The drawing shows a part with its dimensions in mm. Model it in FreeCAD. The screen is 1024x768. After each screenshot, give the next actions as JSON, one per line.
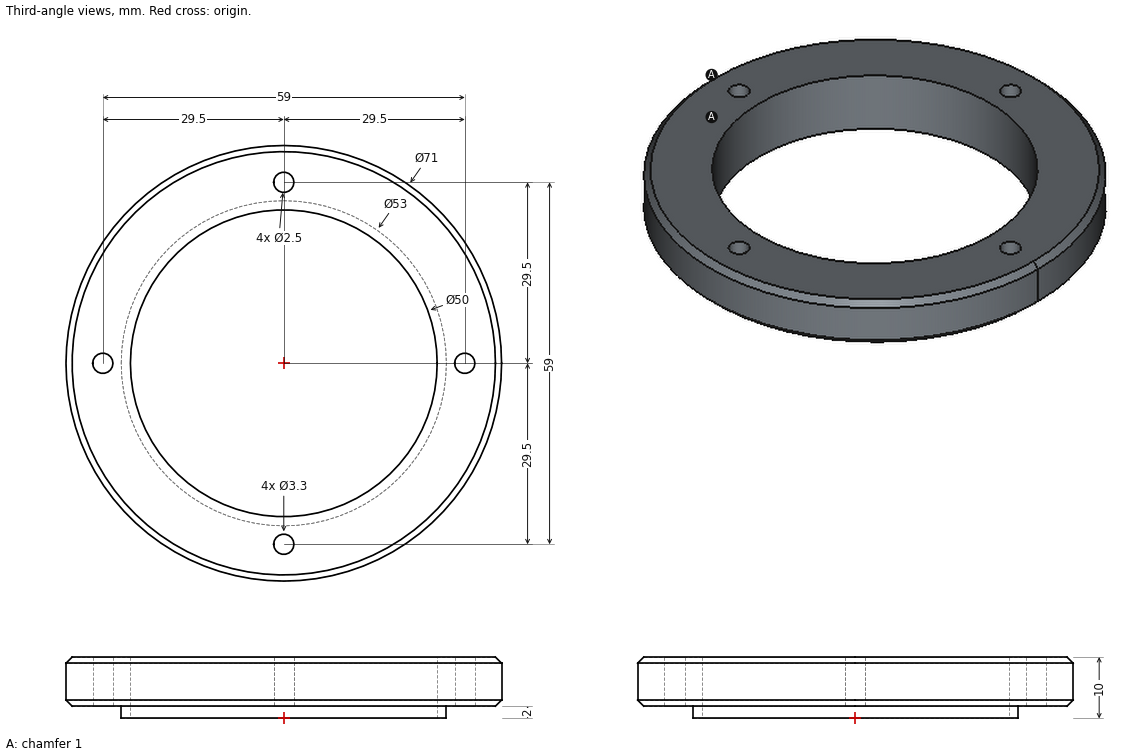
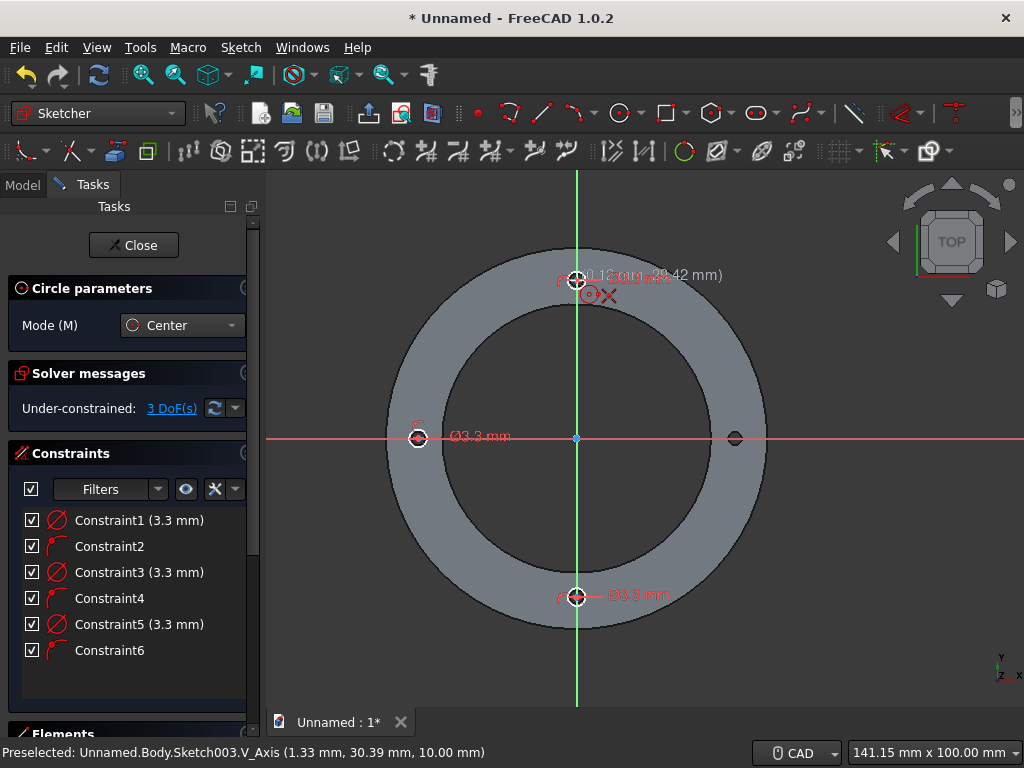
{"action": "scroll", "coordinate": [735, 438], "scroll_direction": "up", "scroll_amount": 5}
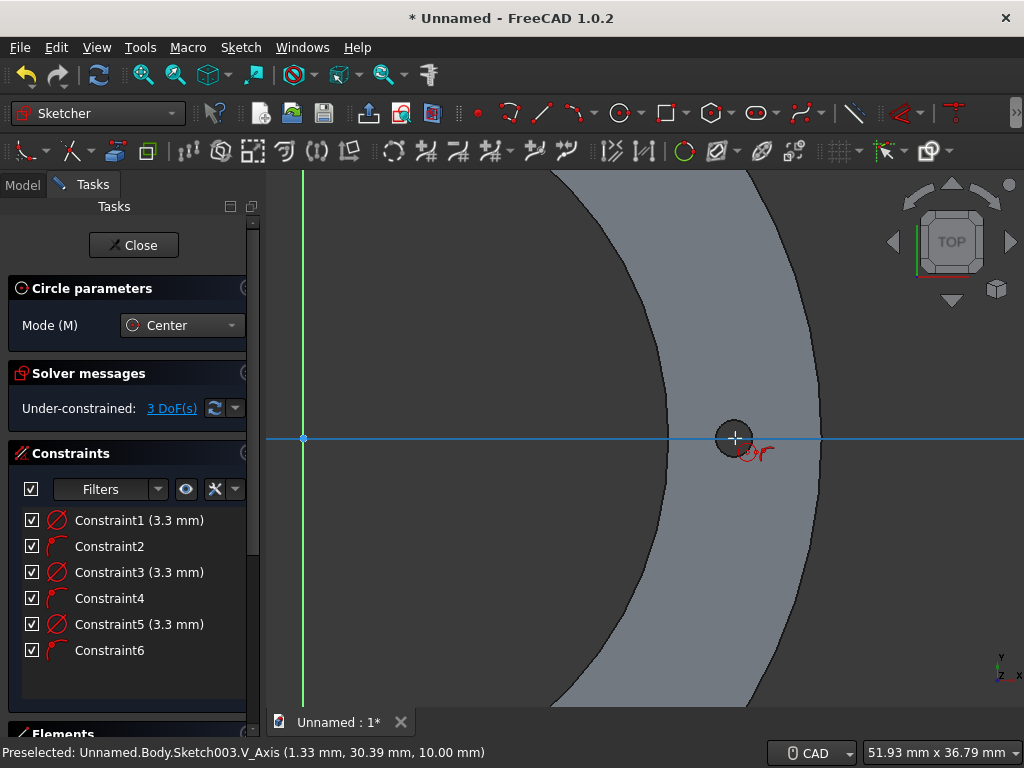
{"action": "left_click", "coordinate": [734, 438]}
{"action": "mouse_move", "coordinate": [751, 421]}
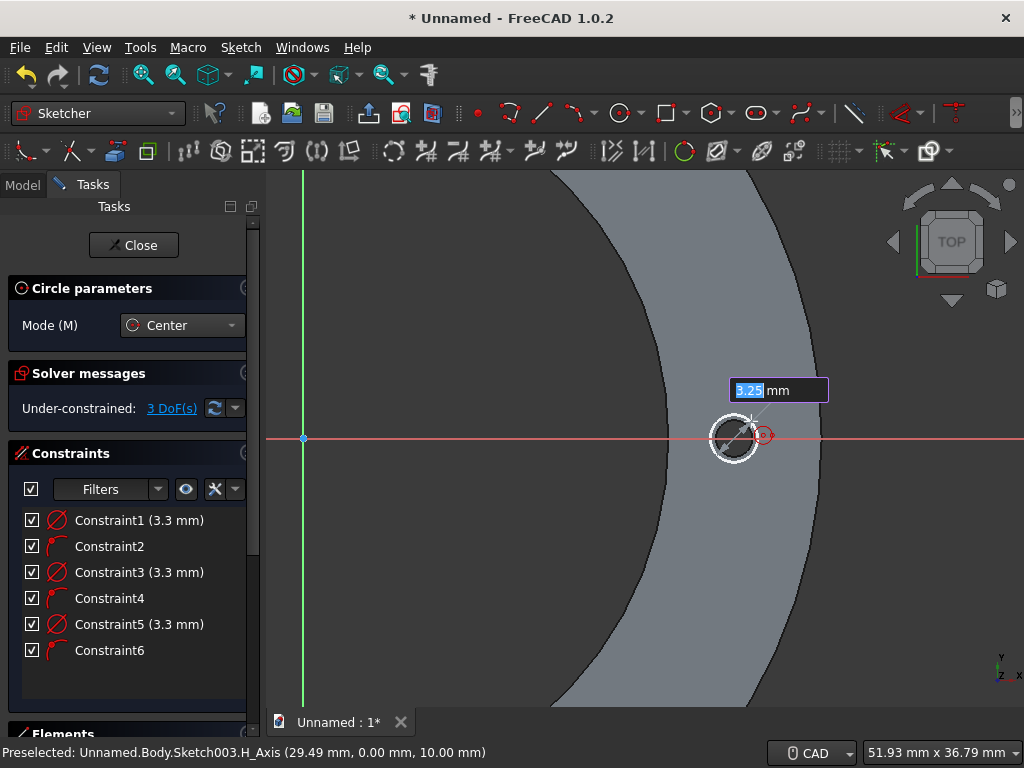
{"action": "type", "text": "3.3"}
{"action": "key", "text": "Return"}
{"action": "key", "text": "Escape"}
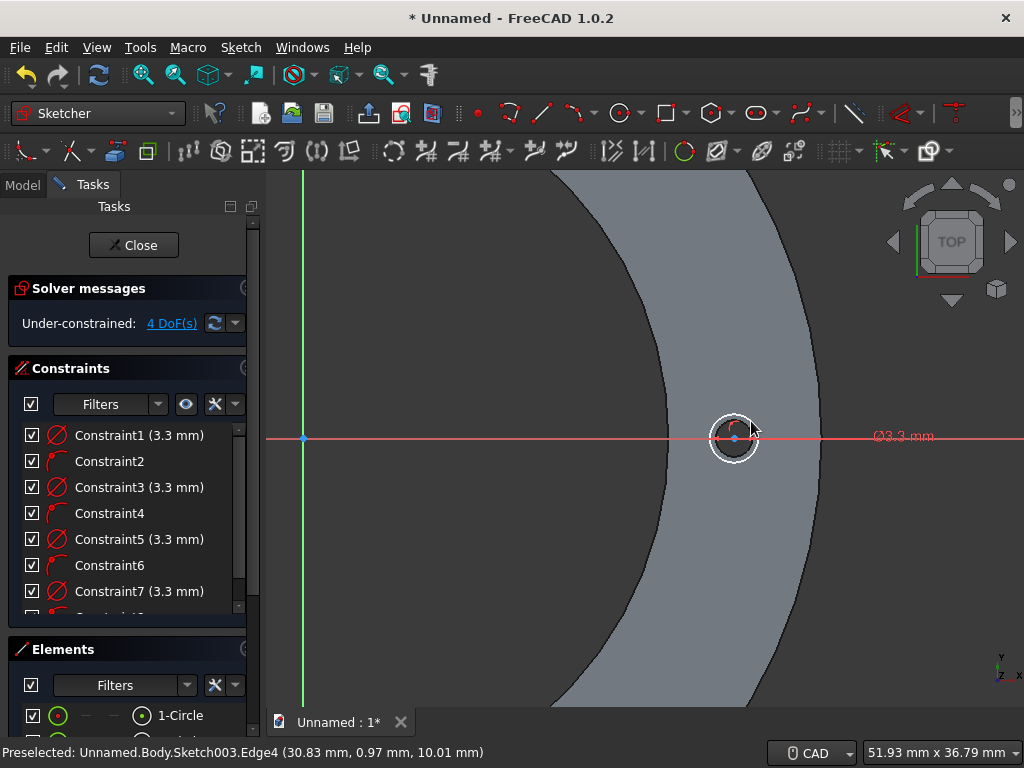
{"action": "scroll", "coordinate": [735, 439], "scroll_direction": "down", "scroll_amount": 5}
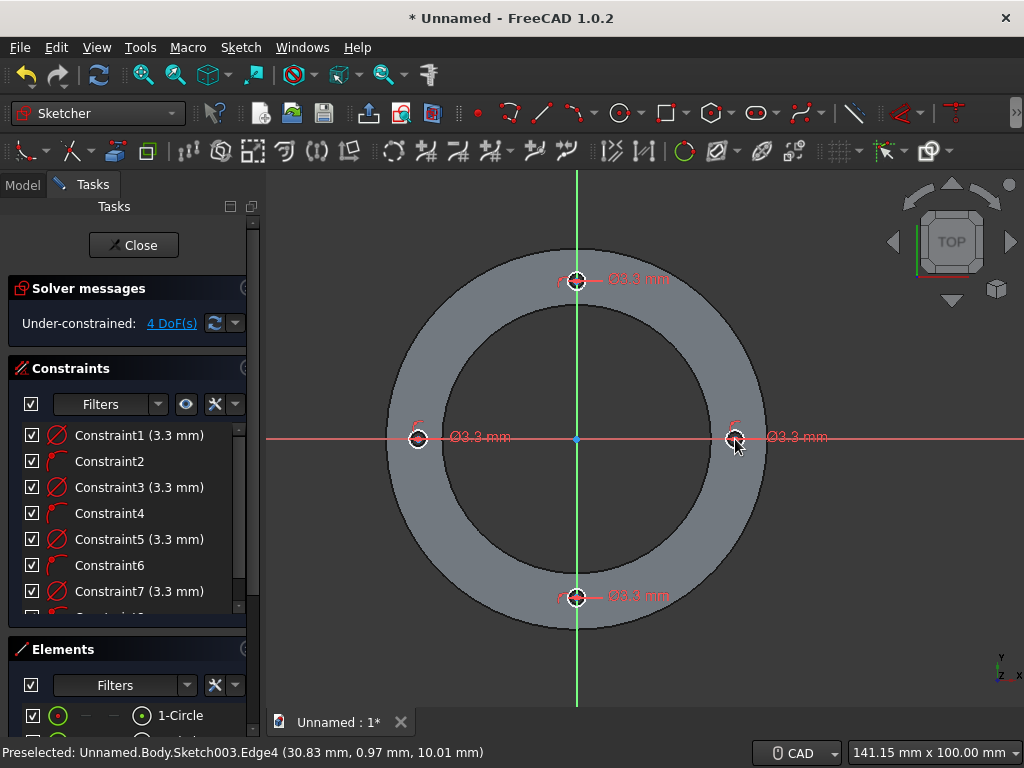
{"action": "left_click", "coordinate": [577, 598]}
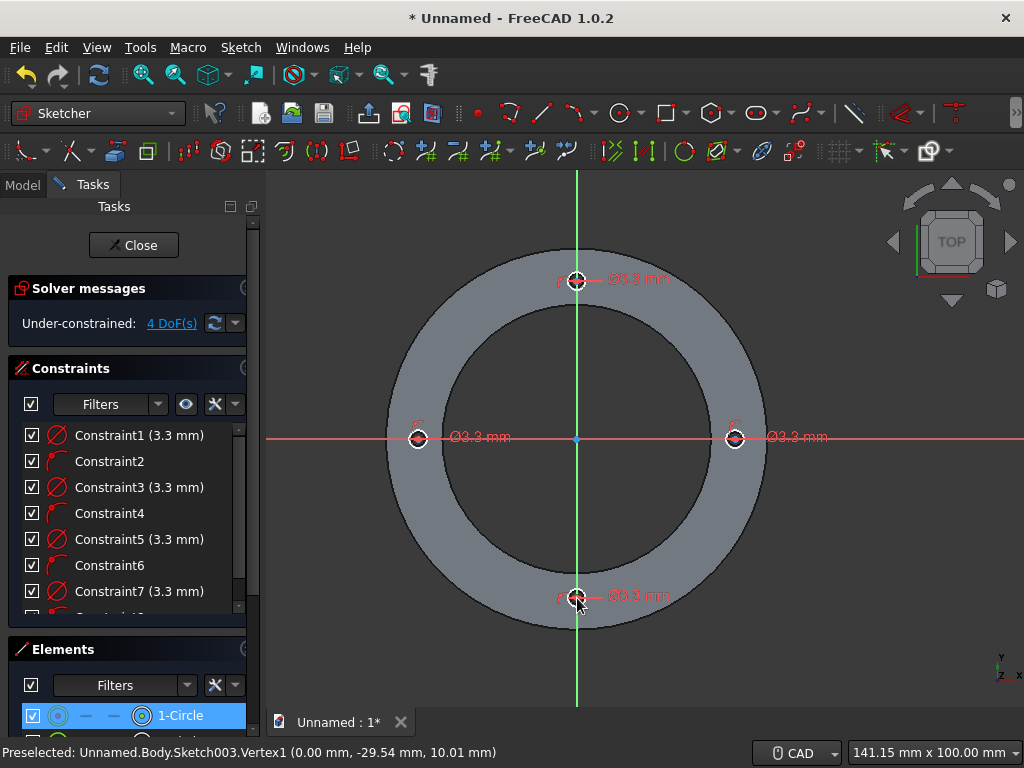
{"action": "left_click", "coordinate": [577, 281]}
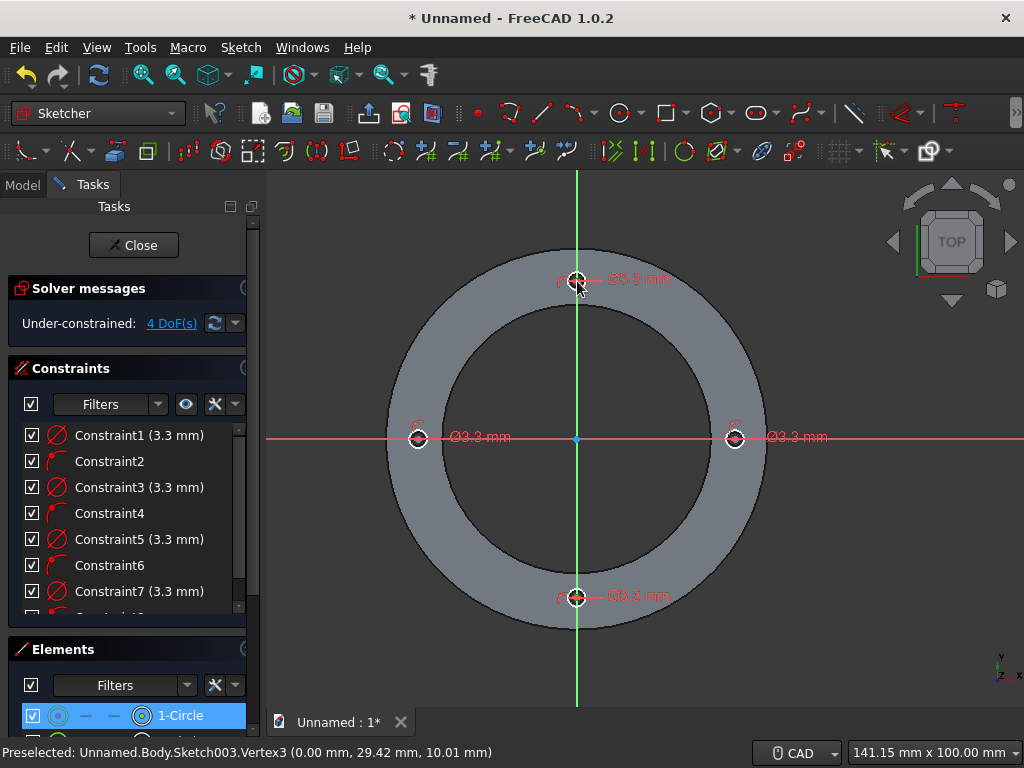
{"action": "key", "text": "i"}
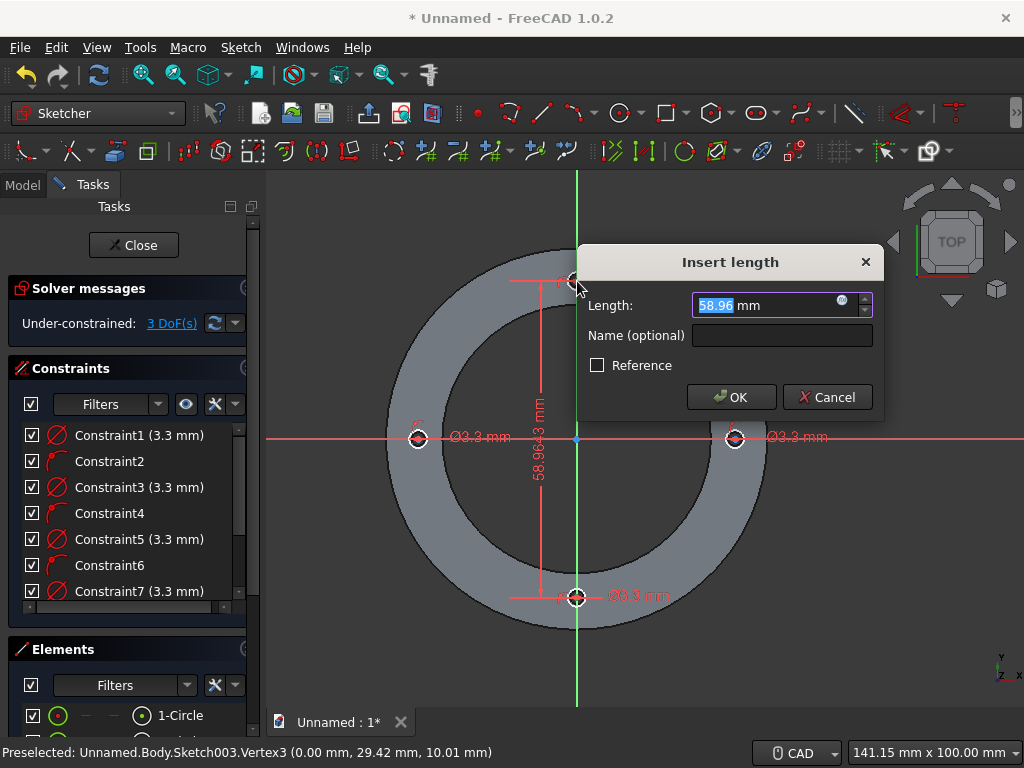
{"action": "type", "text": "59"}
{"action": "key", "text": "Return"}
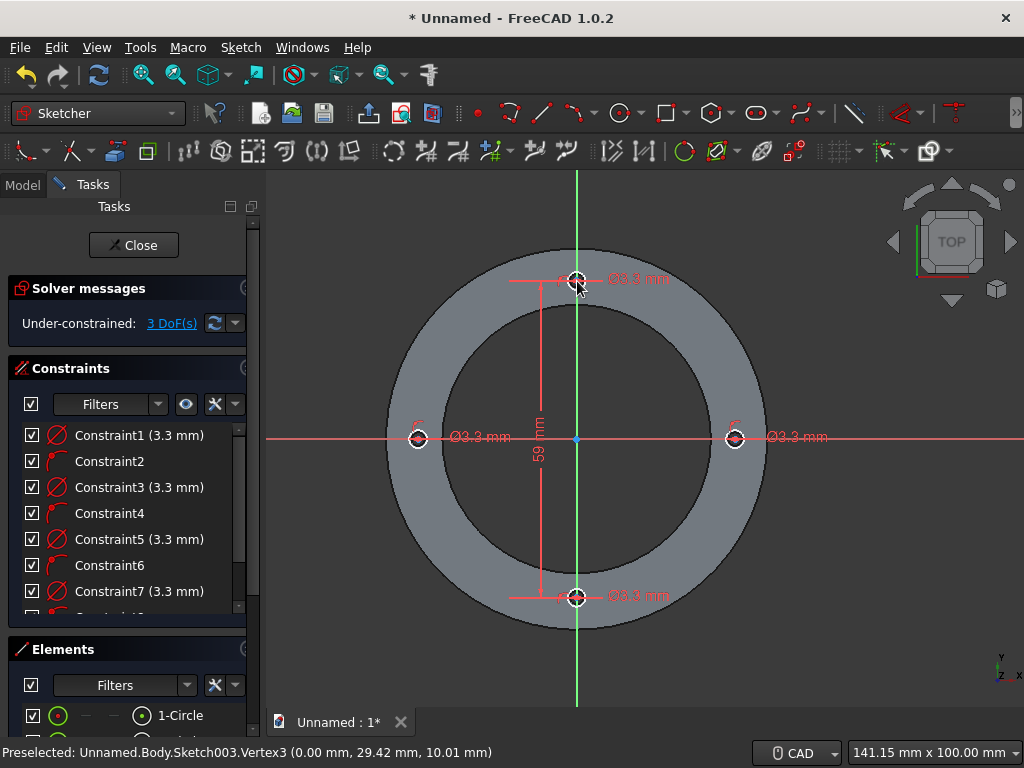
{"action": "left_click", "coordinate": [418, 439]}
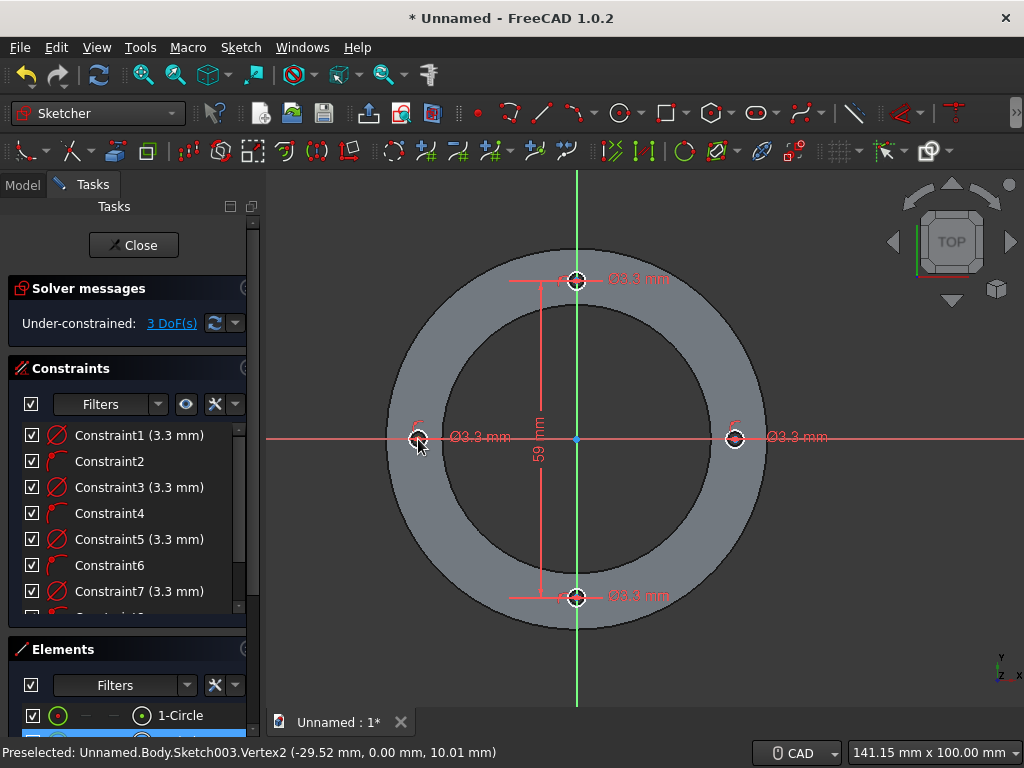
{"action": "left_click", "coordinate": [735, 439]}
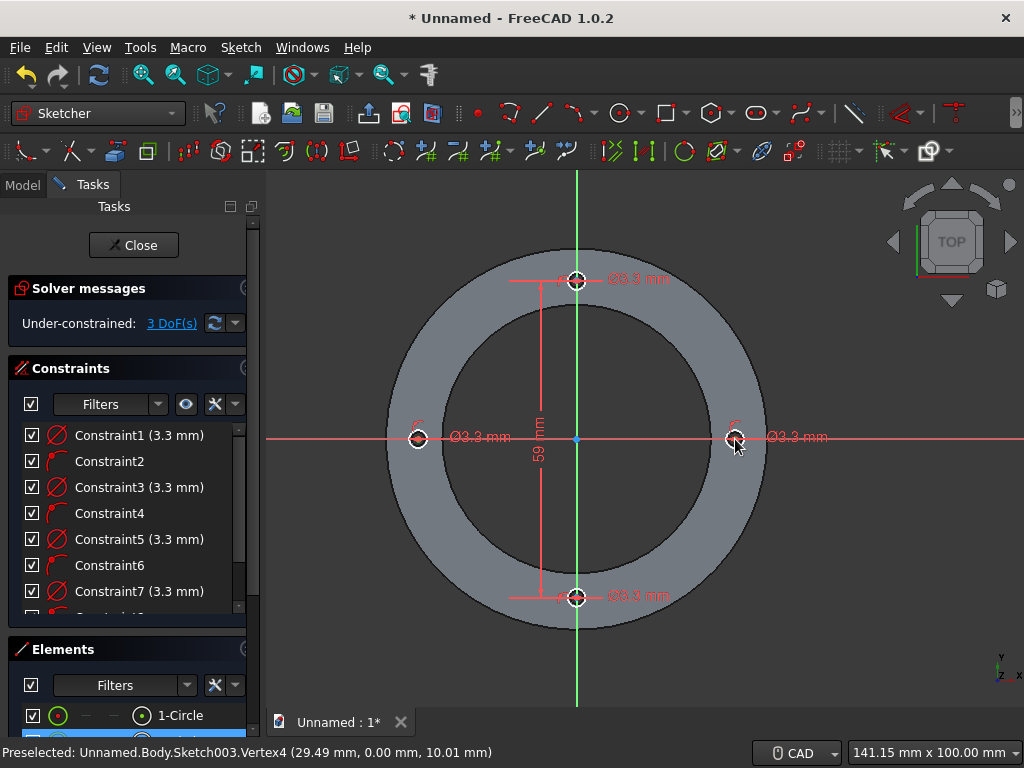
{"action": "key", "text": "l"}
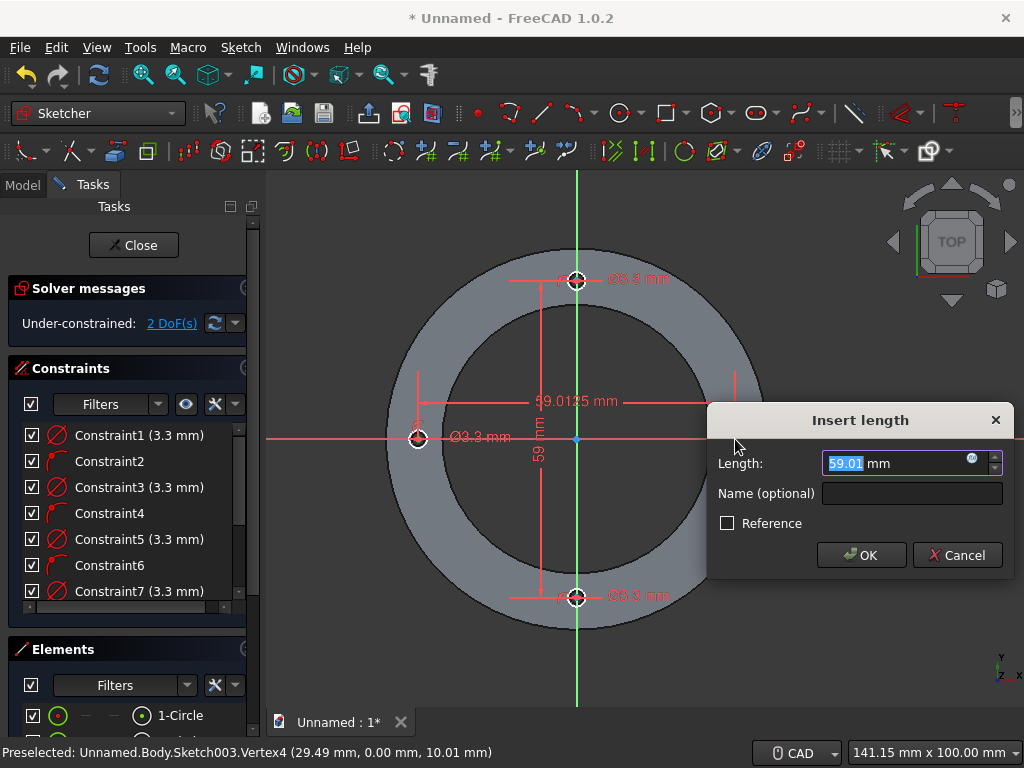
{"action": "type", "text": "59"}
{"action": "key", "text": "Return"}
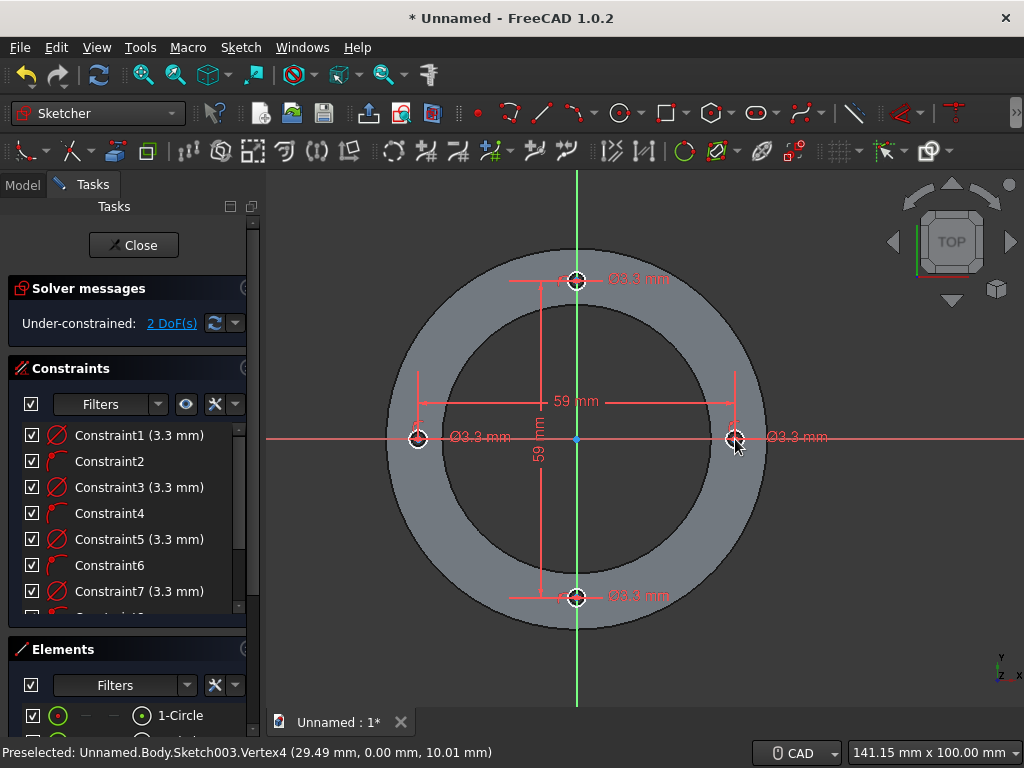
{"action": "left_click", "coordinate": [577, 598]}